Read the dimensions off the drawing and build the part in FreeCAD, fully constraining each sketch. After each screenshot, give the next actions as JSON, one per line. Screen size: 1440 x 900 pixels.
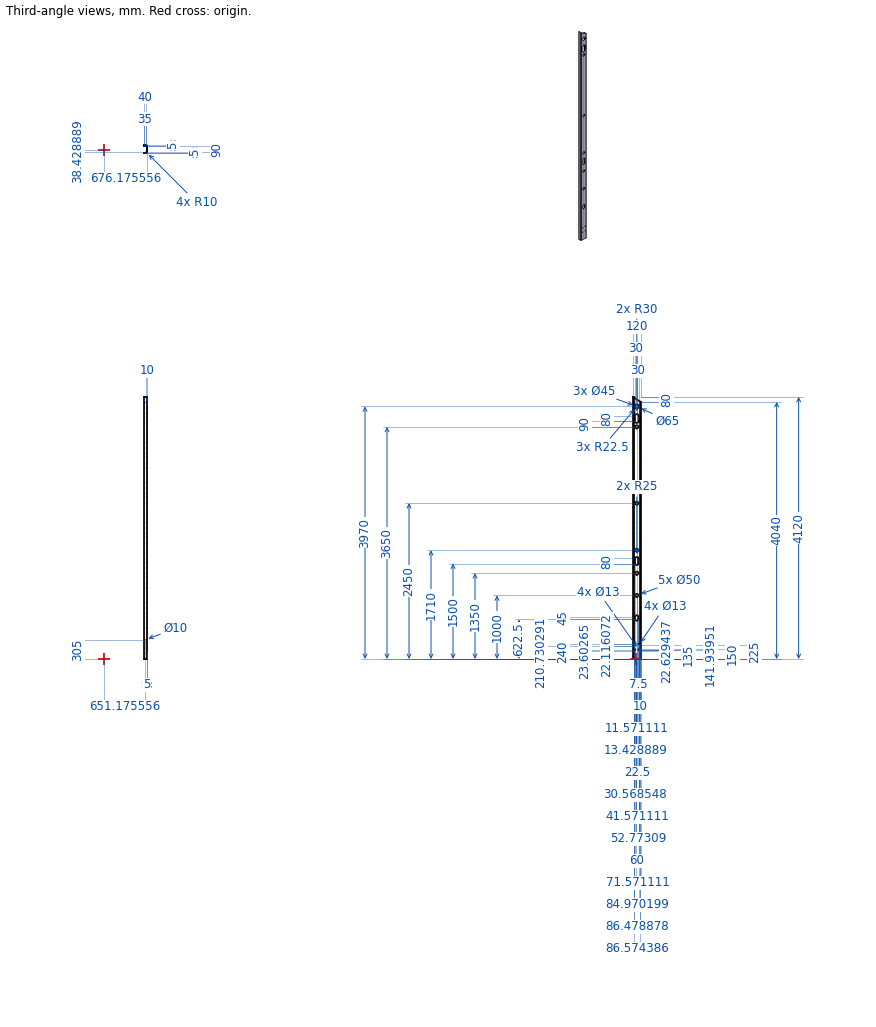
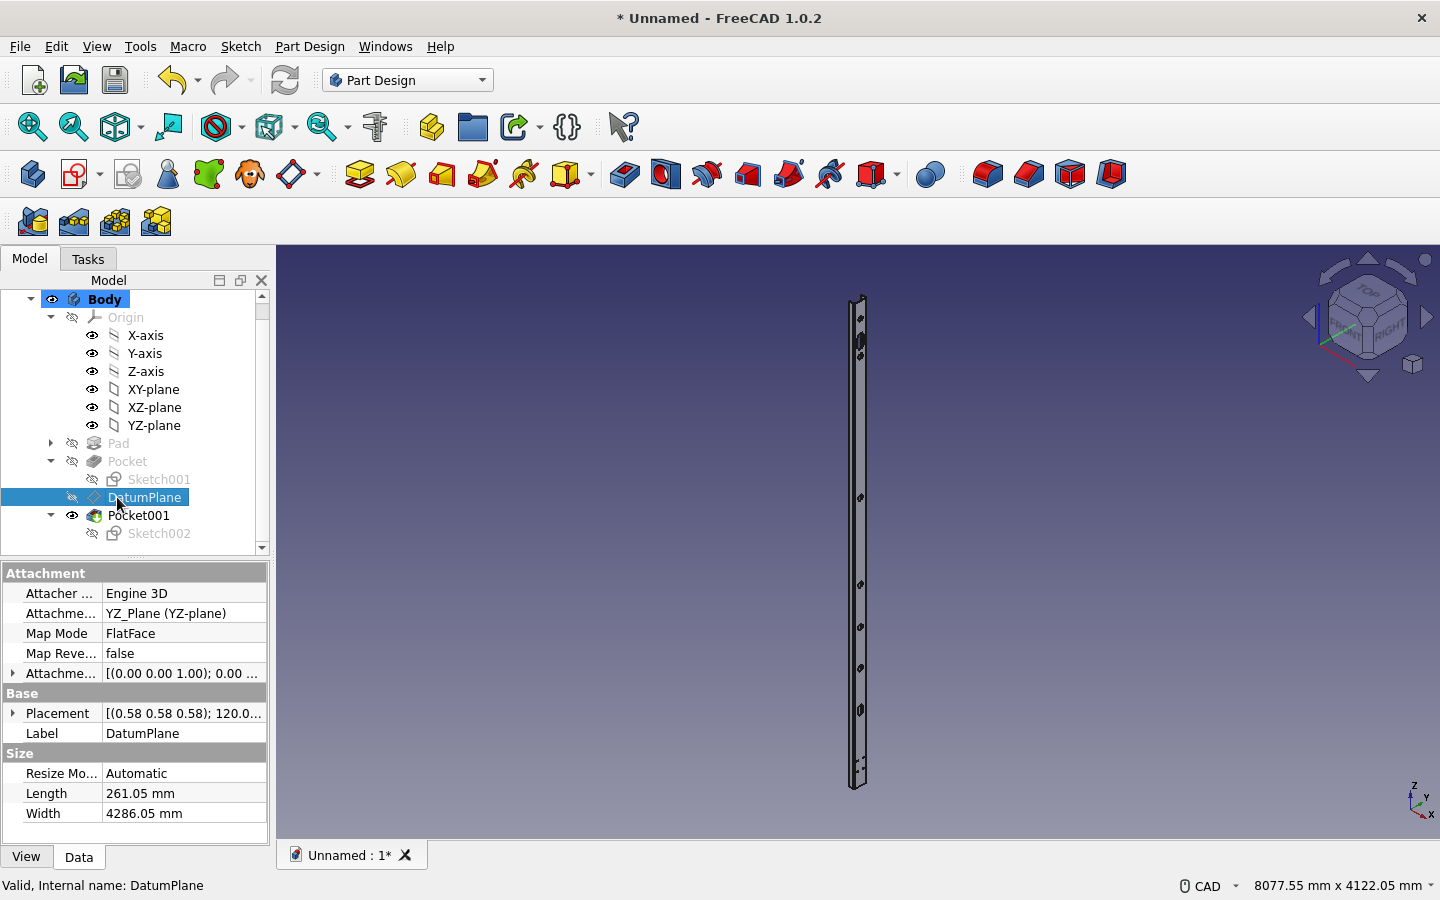
{"action": "key", "text": "3"}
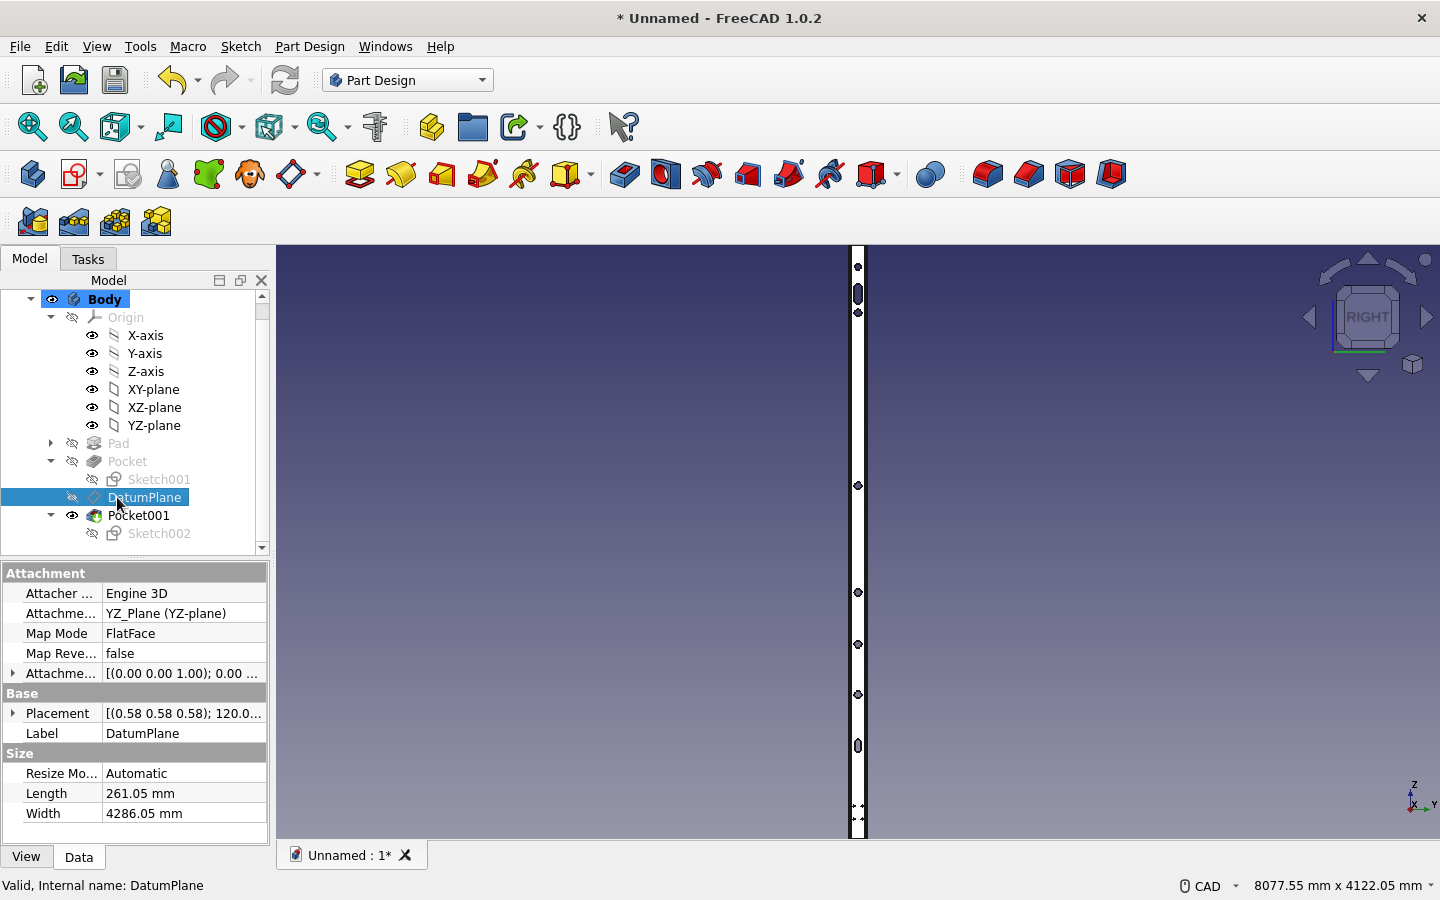
{"action": "left_click", "coordinate": [33, 128]}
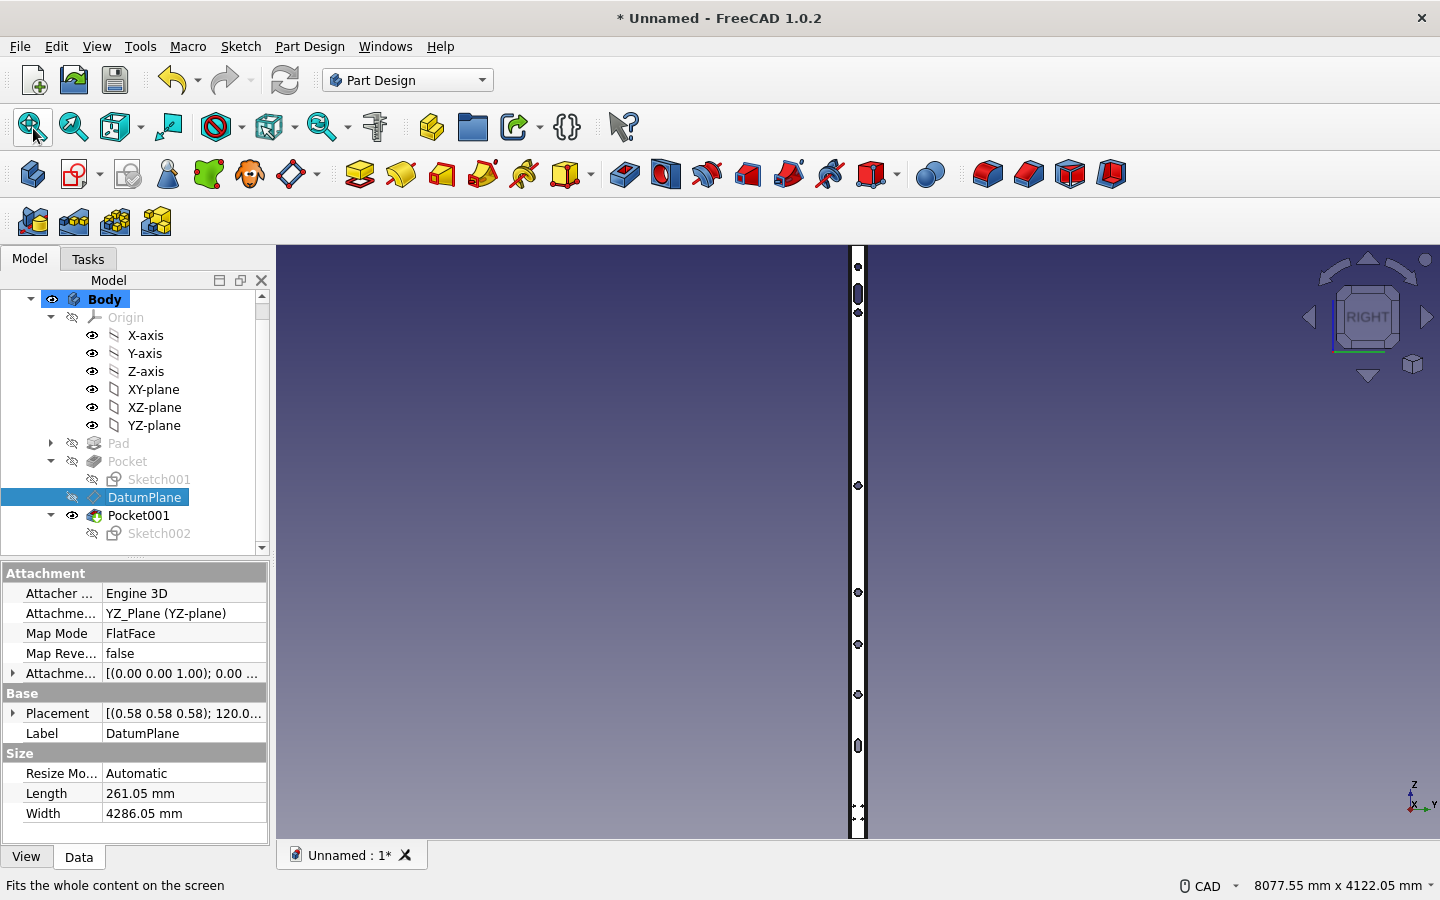
{"action": "key", "text": "2"}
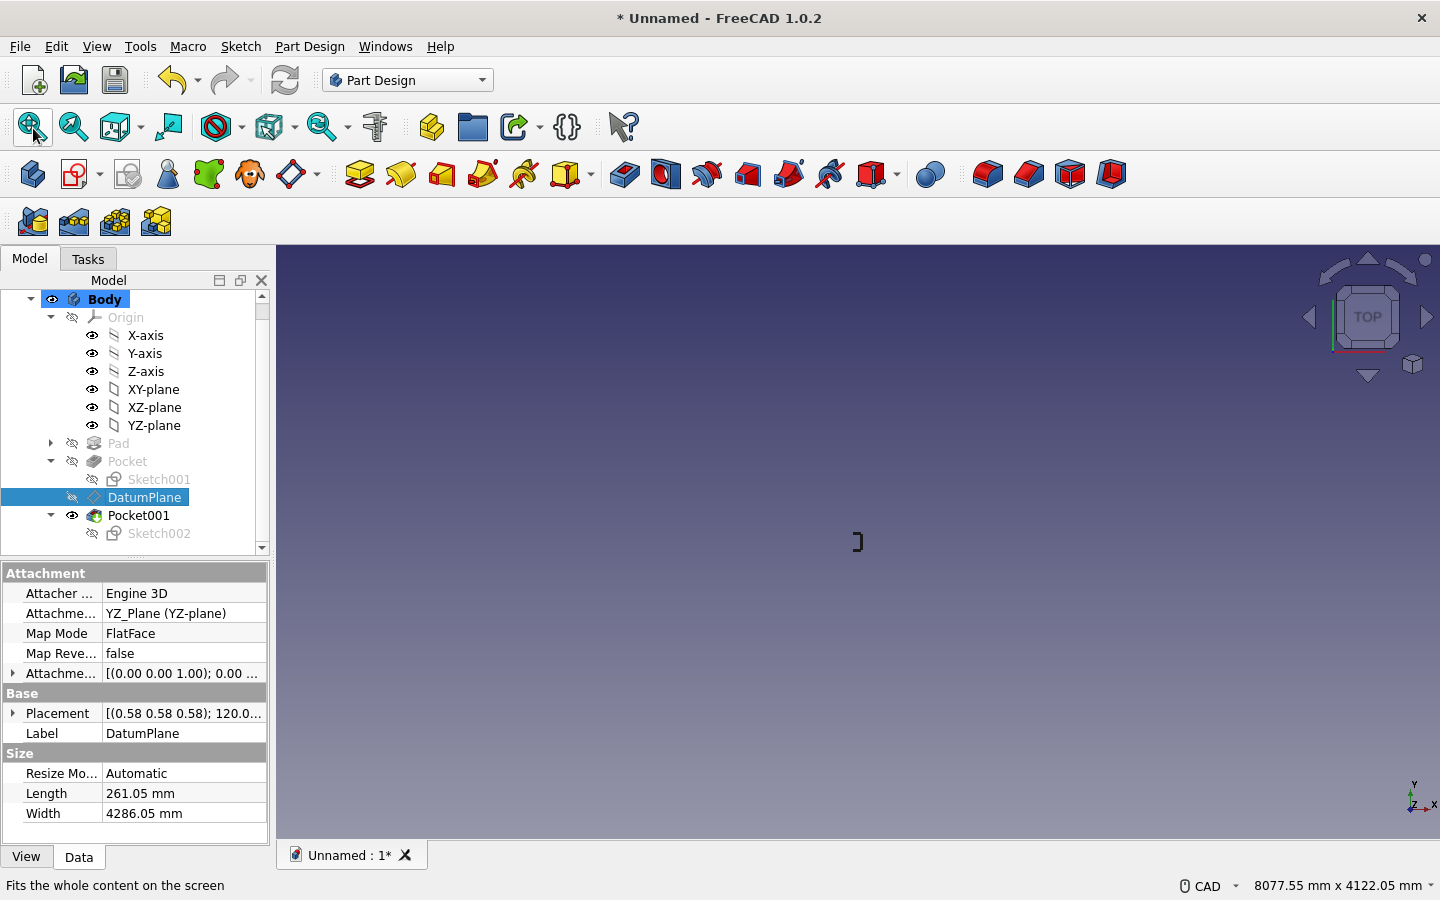
{"action": "left_click", "coordinate": [33, 128]}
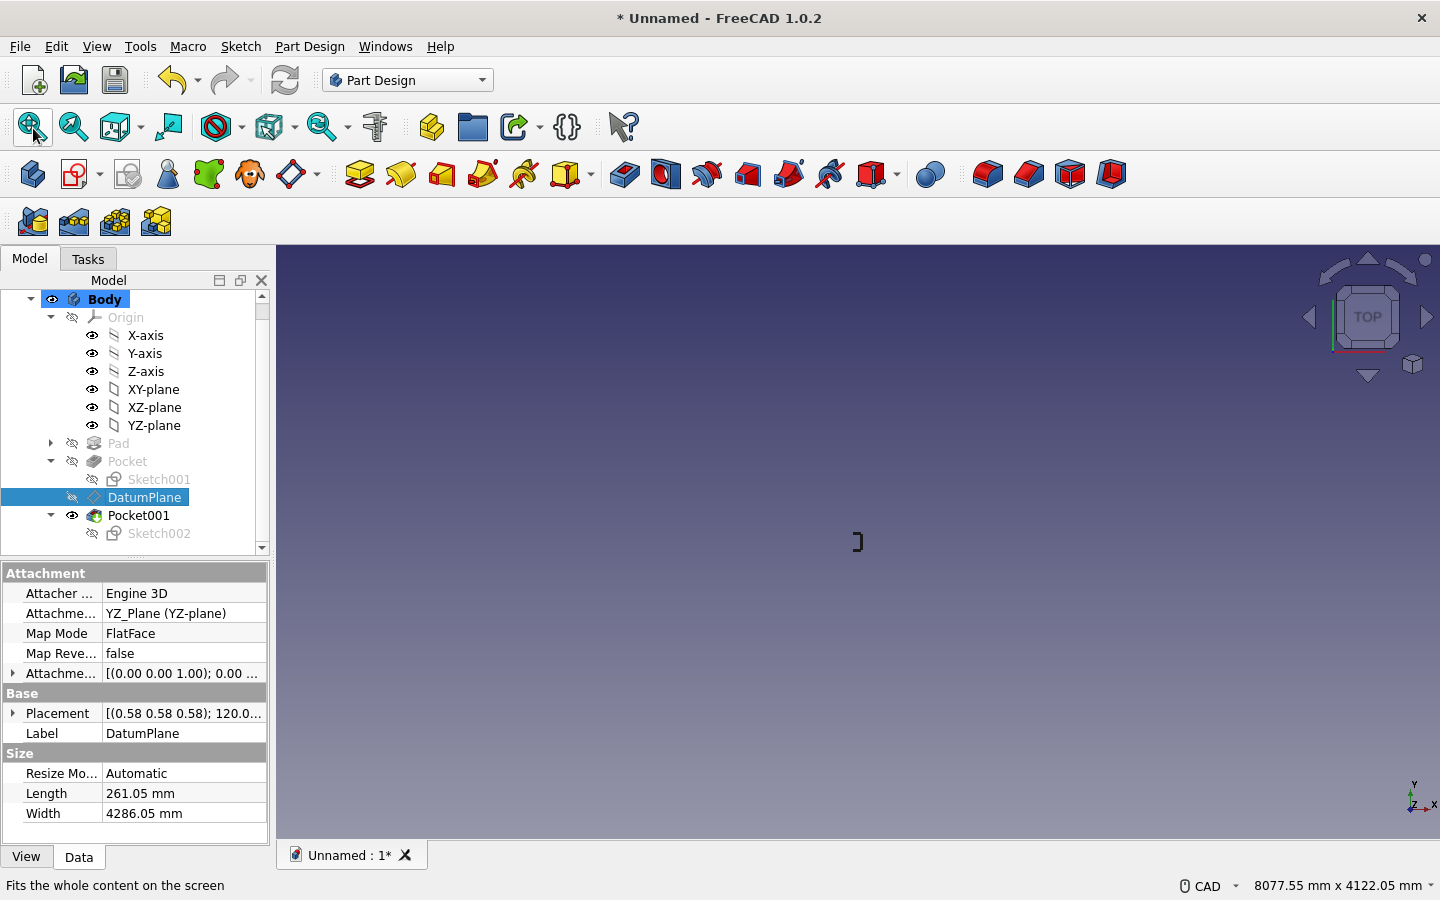
{"action": "left_click", "coordinate": [137, 425]}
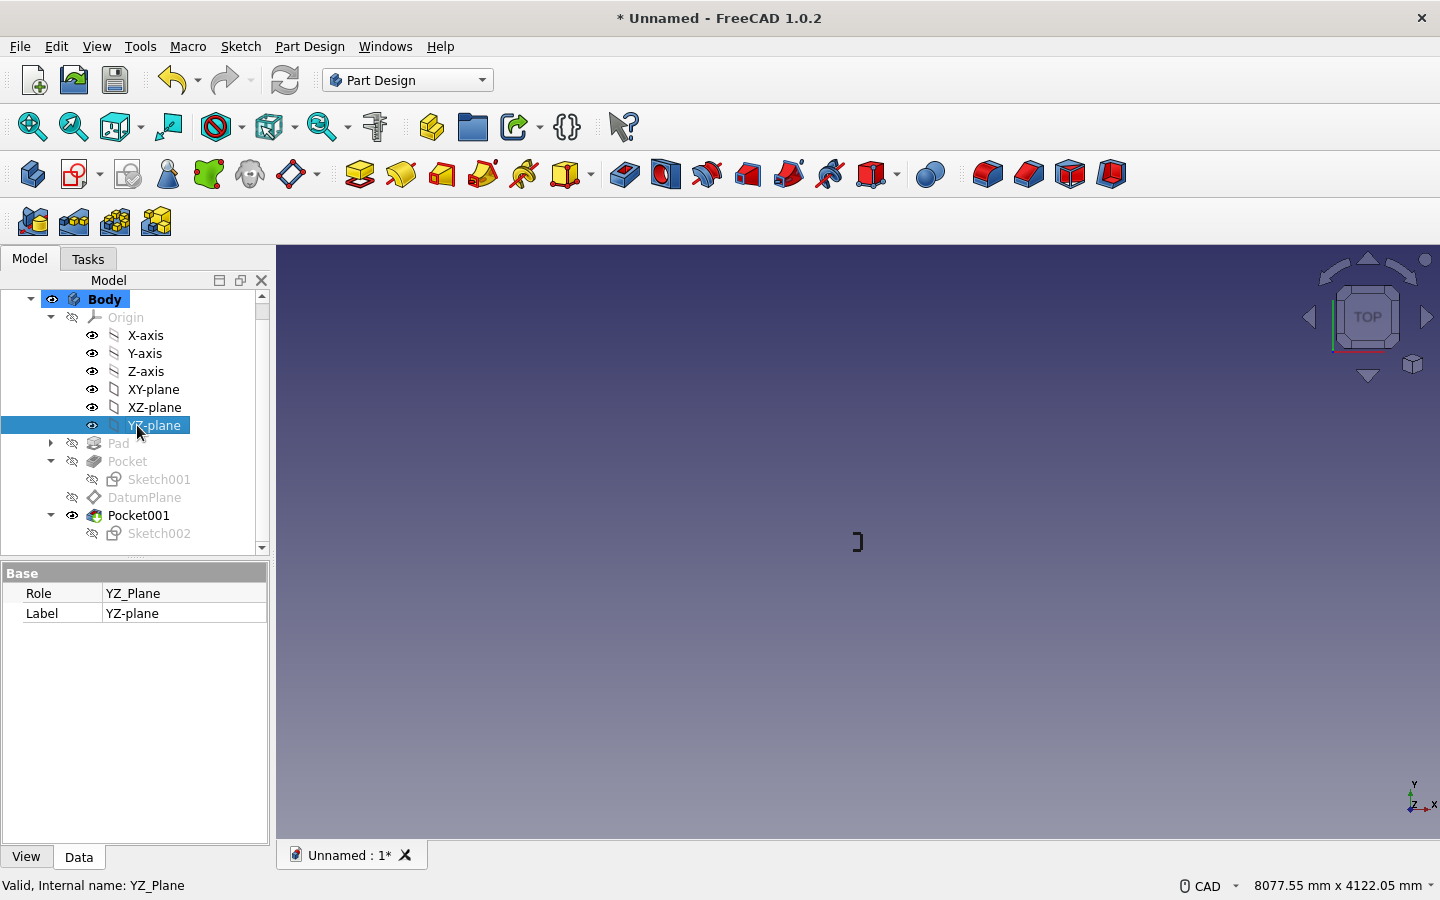
{"action": "left_click", "coordinate": [290, 174]}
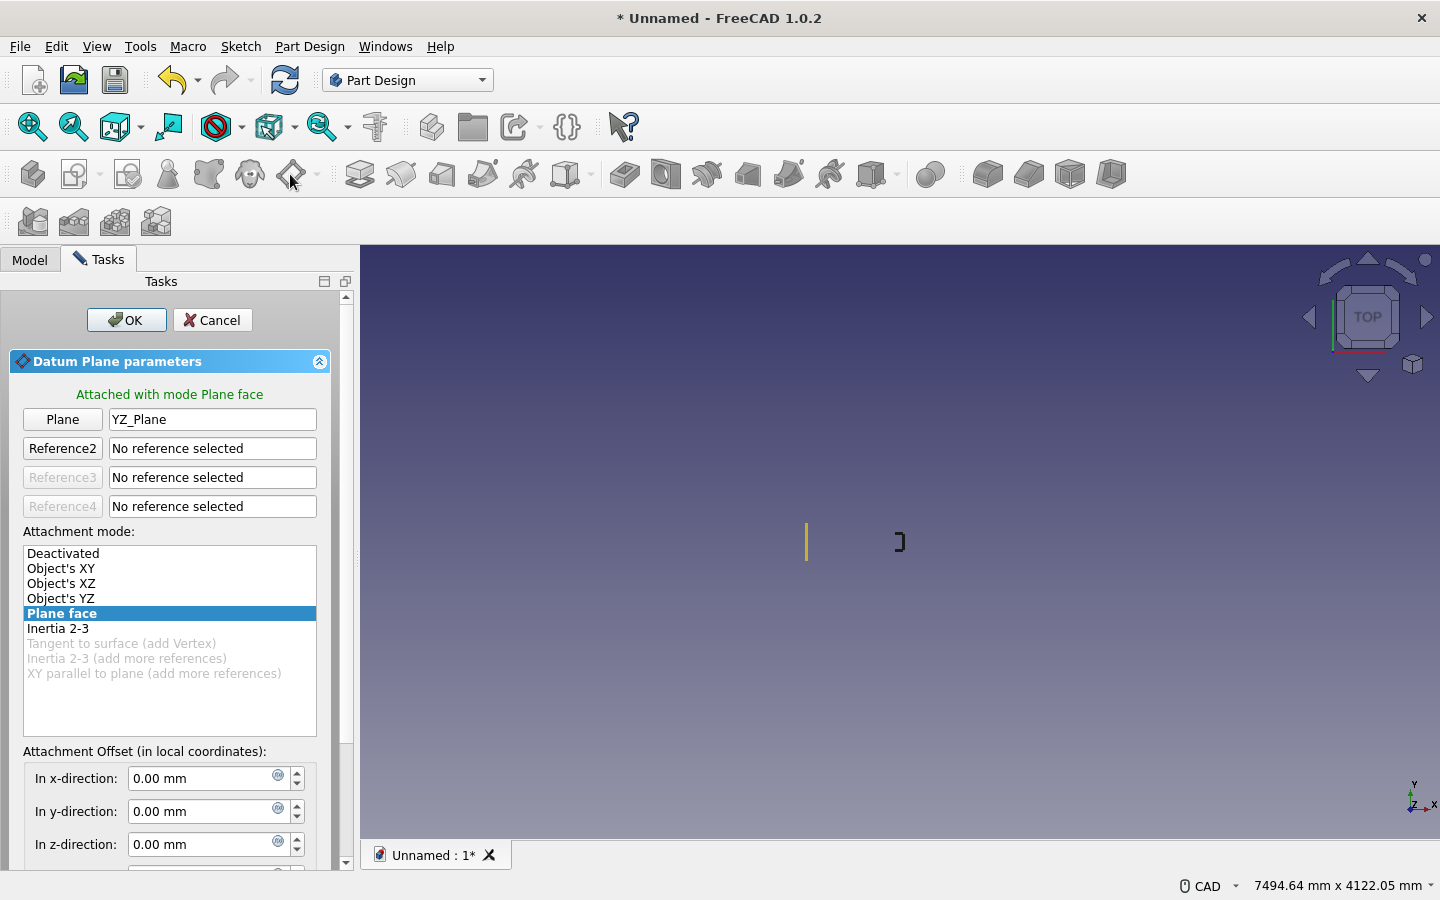
{"action": "triple_click", "coordinate": [210, 844]}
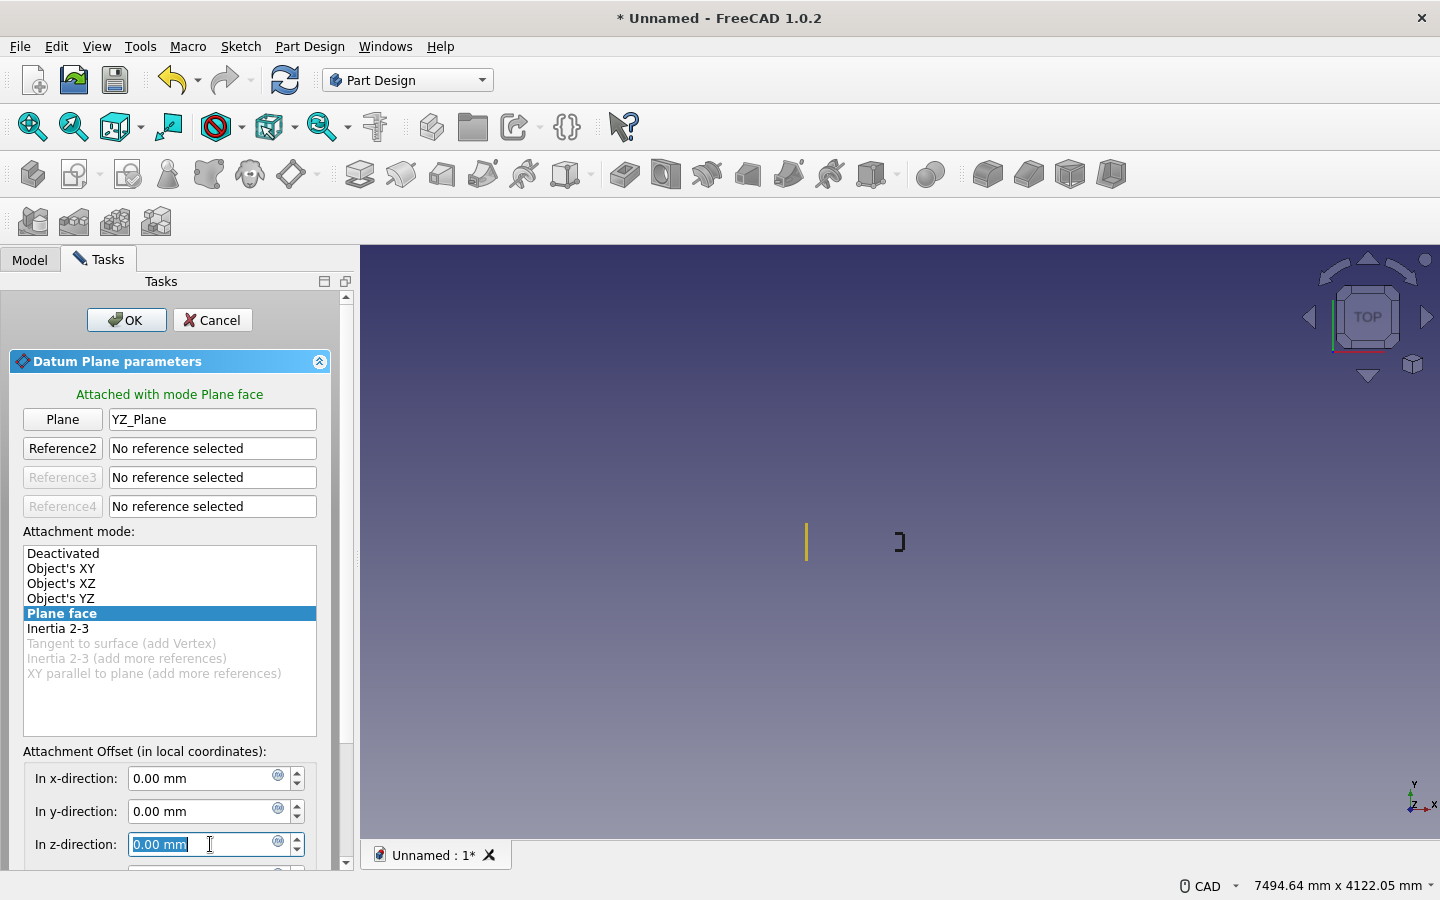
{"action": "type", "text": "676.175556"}
{"action": "key", "text": "Tab"}